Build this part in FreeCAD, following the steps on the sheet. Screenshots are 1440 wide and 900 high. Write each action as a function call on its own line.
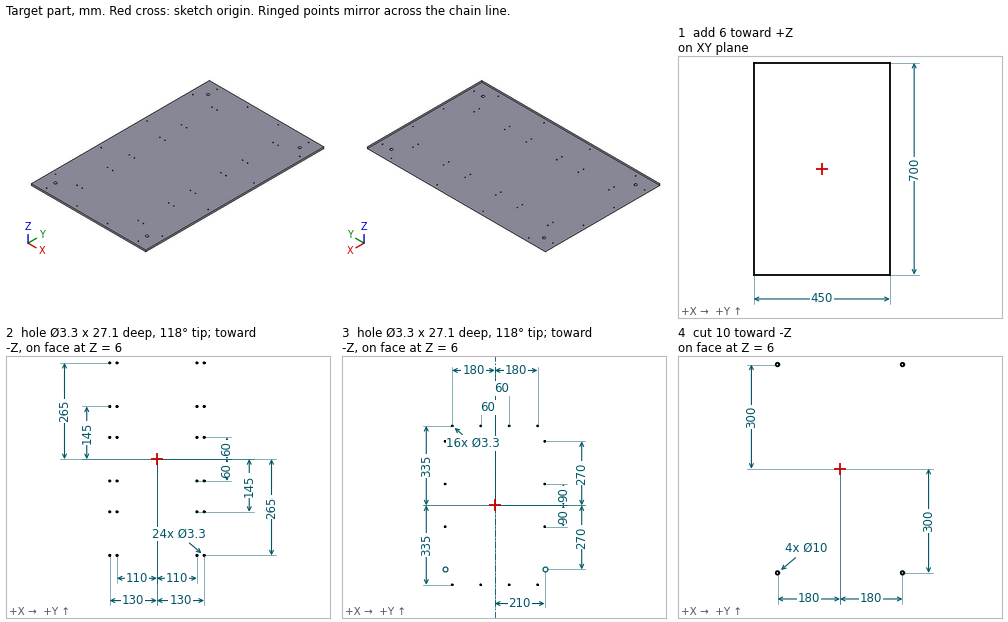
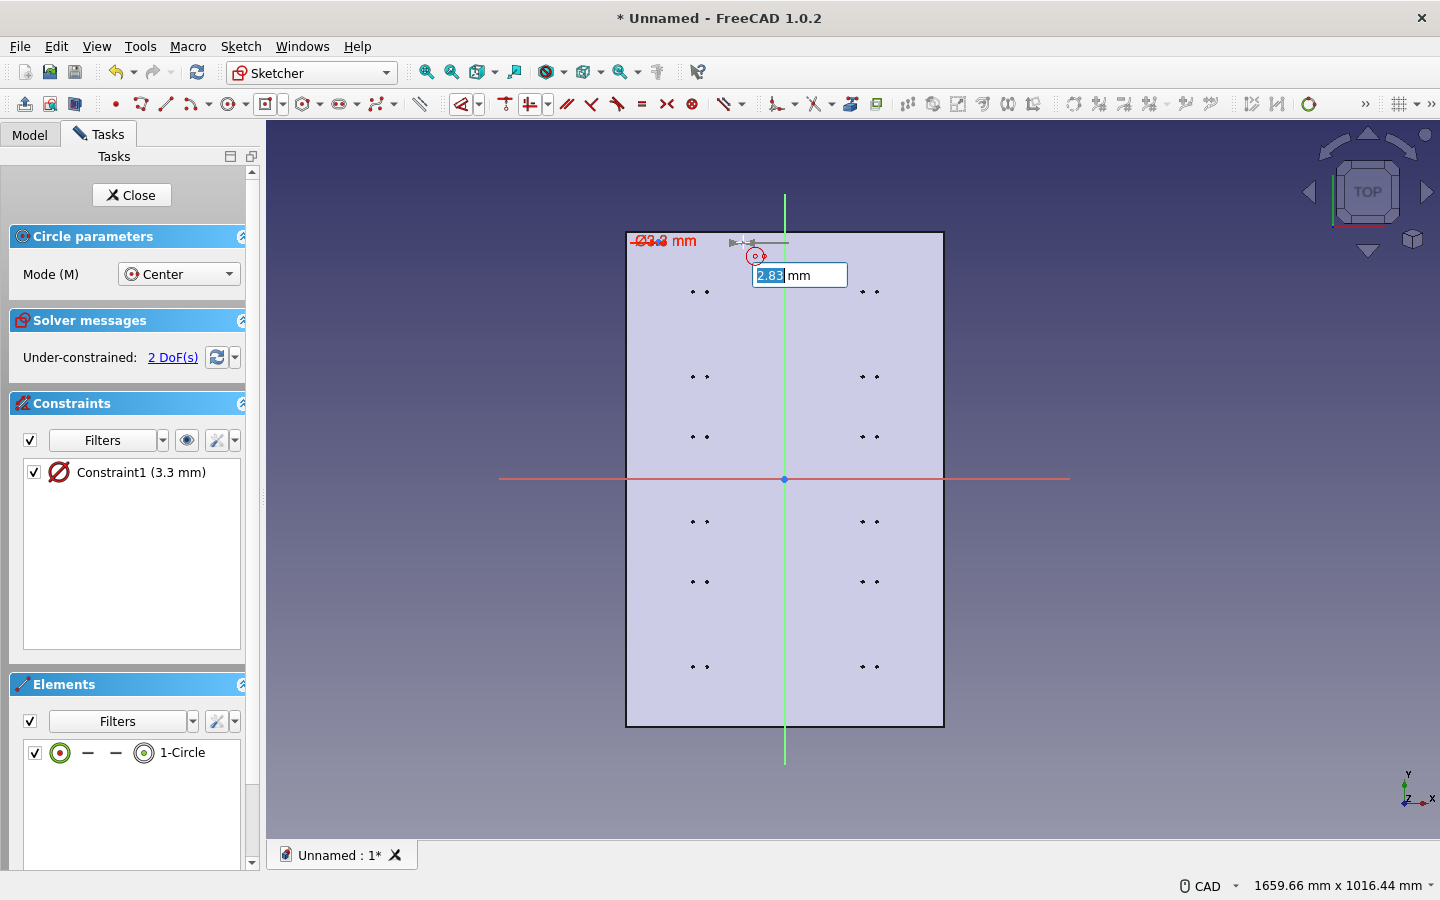
text(3.3)
key(Return)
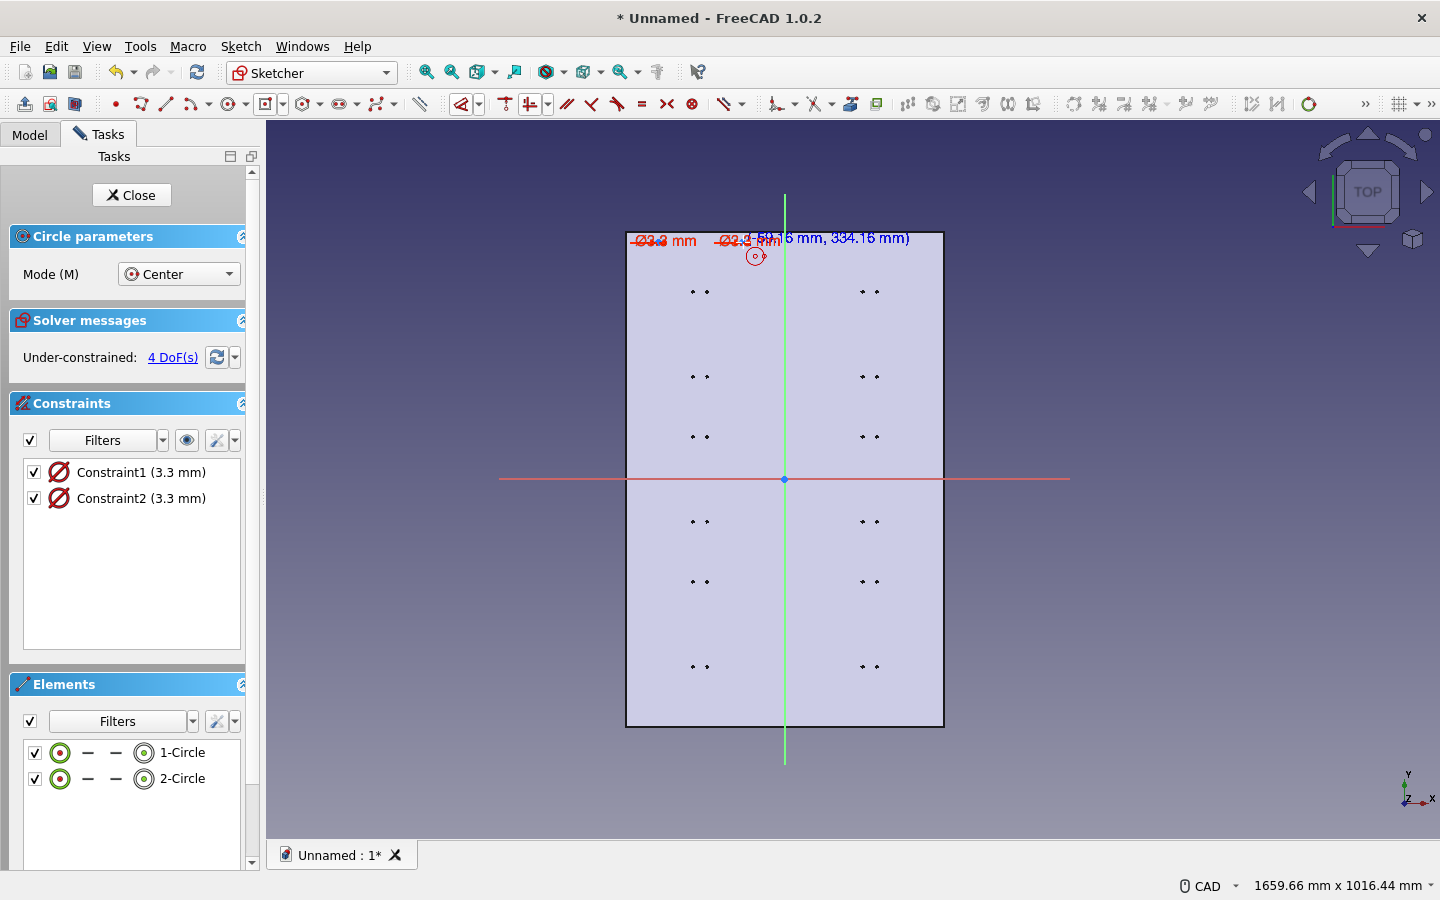
scroll(827, 242, up, 15)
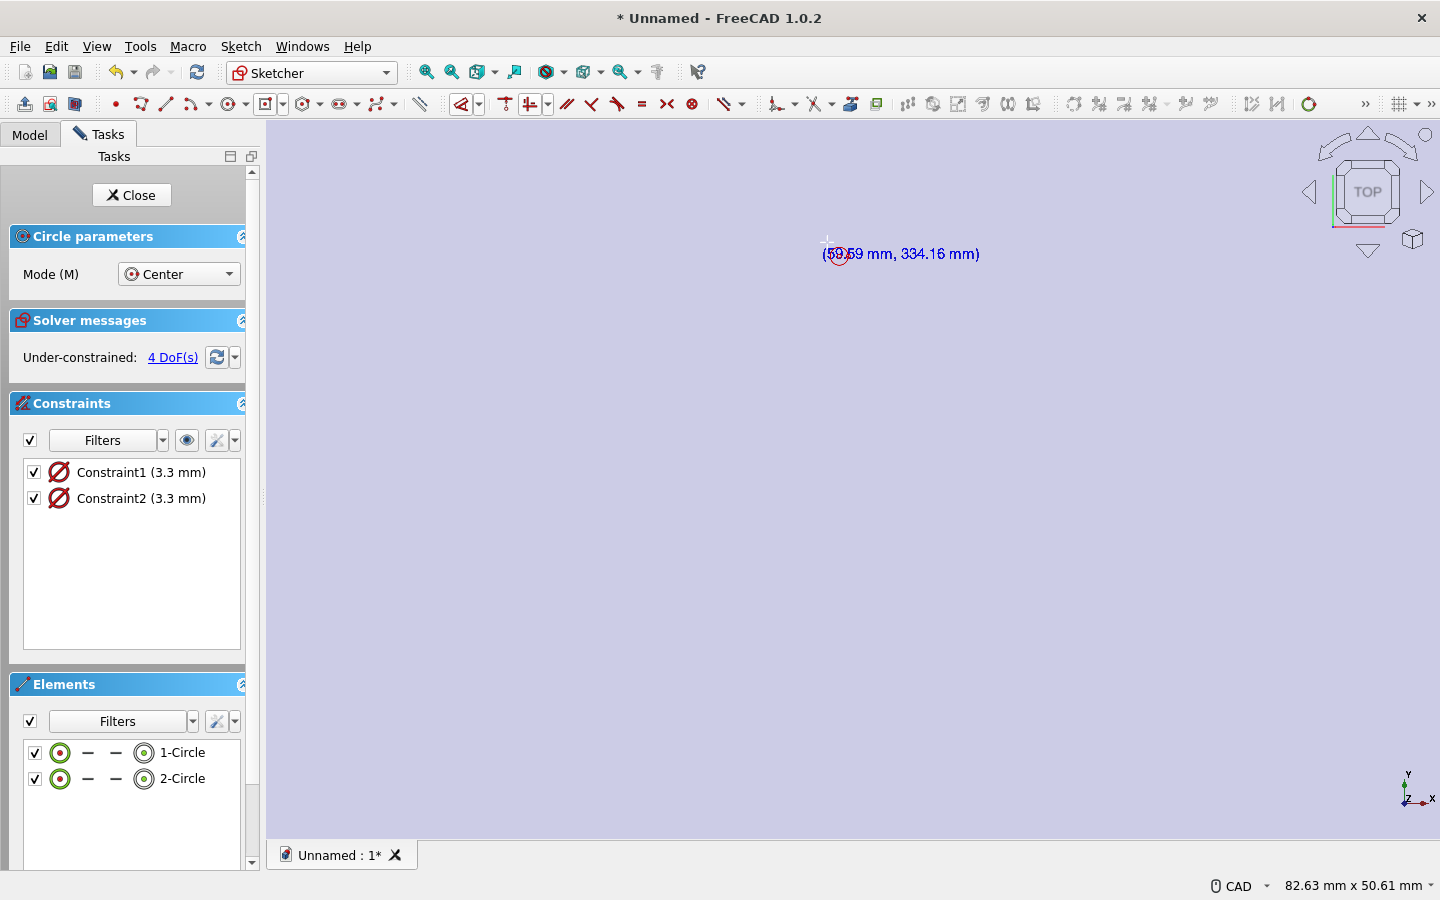
scroll(827, 242, down, 15)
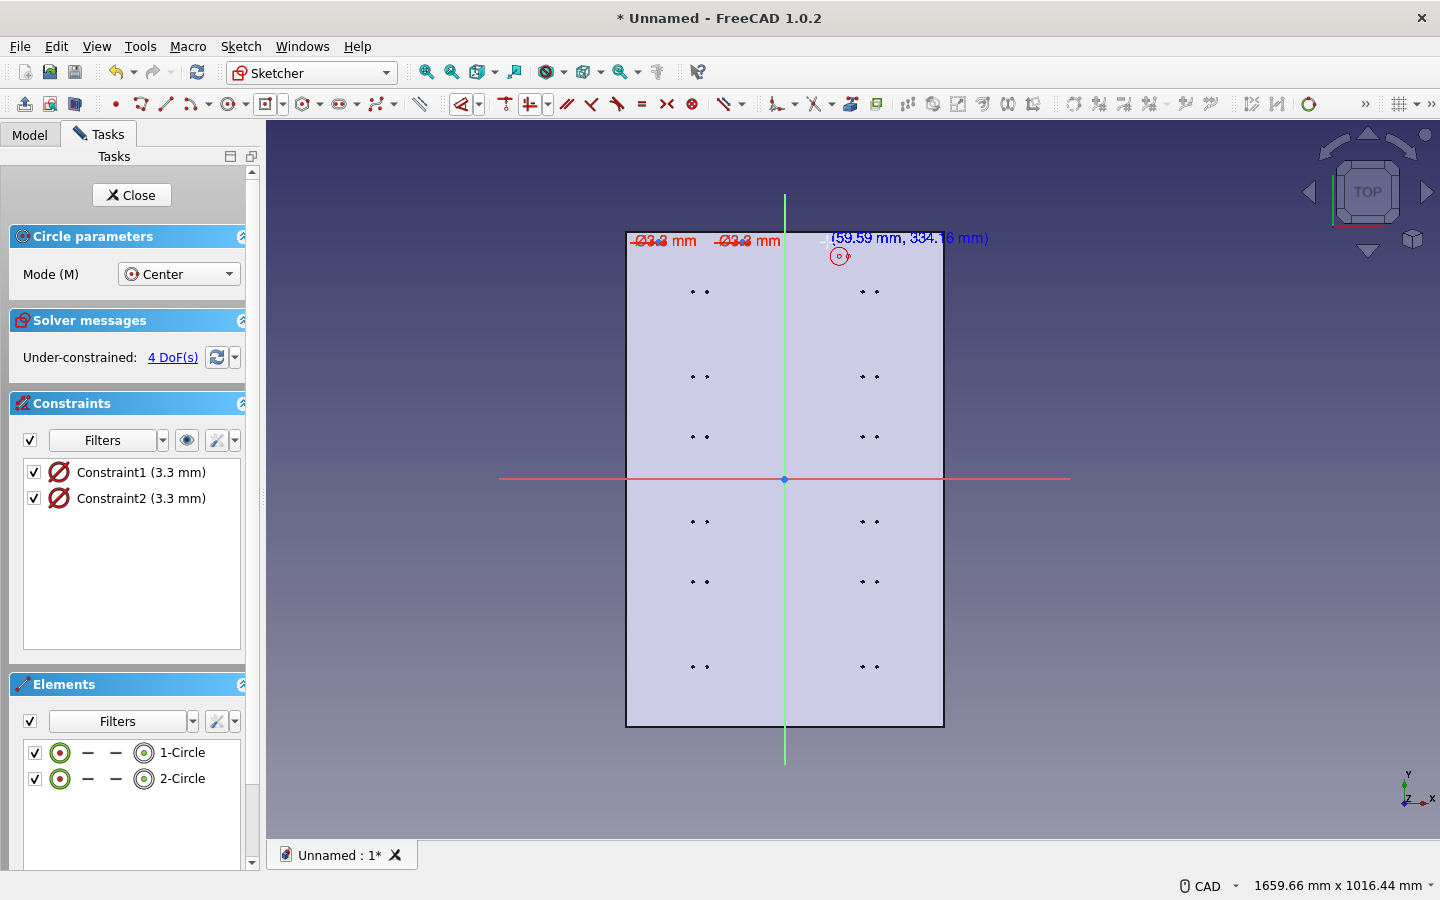
click(827, 242)
move(828, 242)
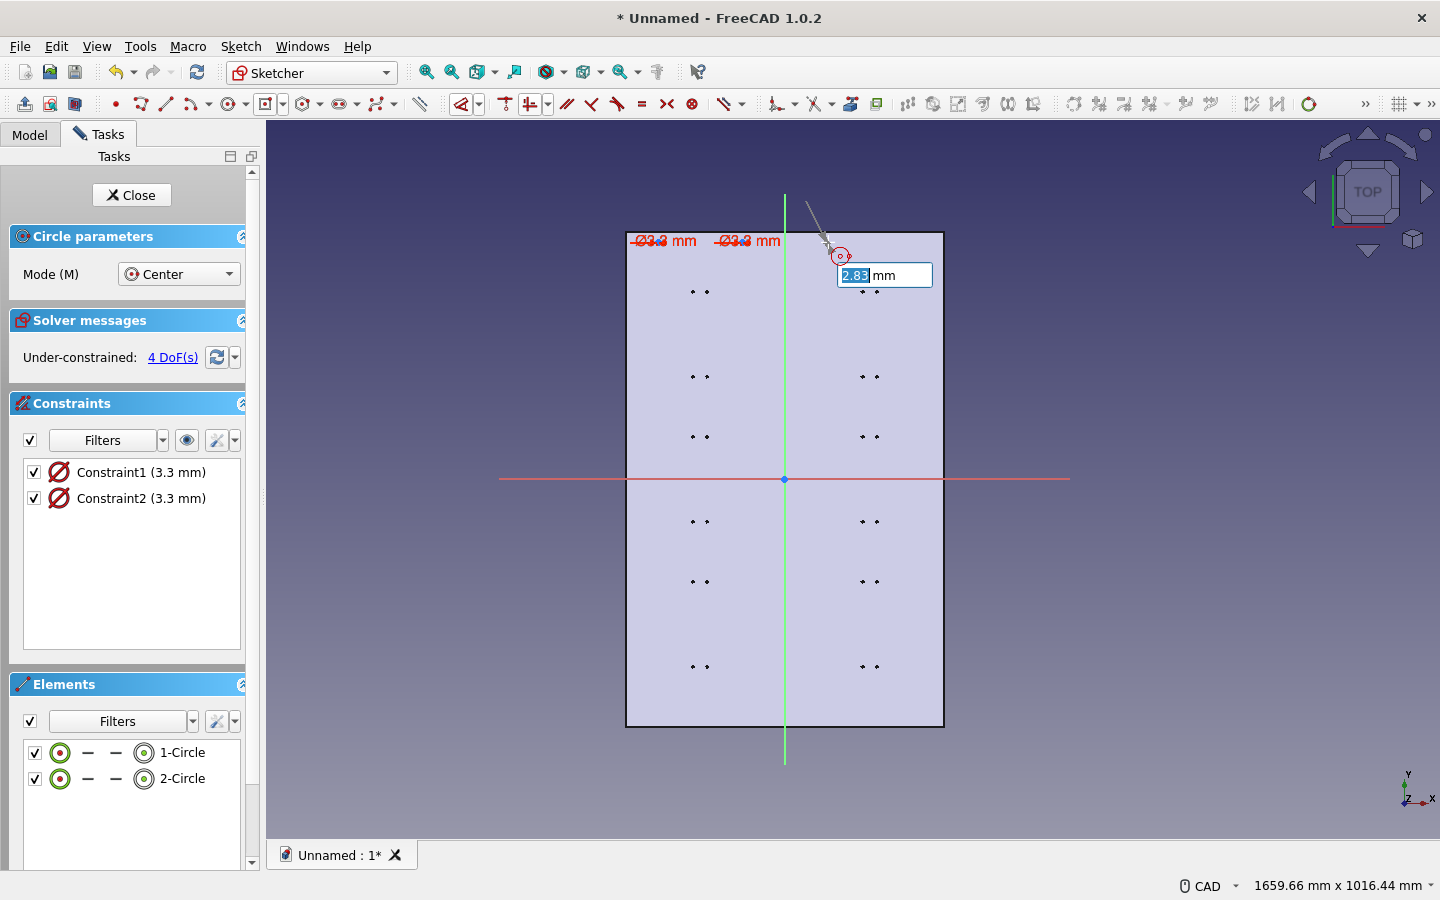
text(3.3)
key(Return)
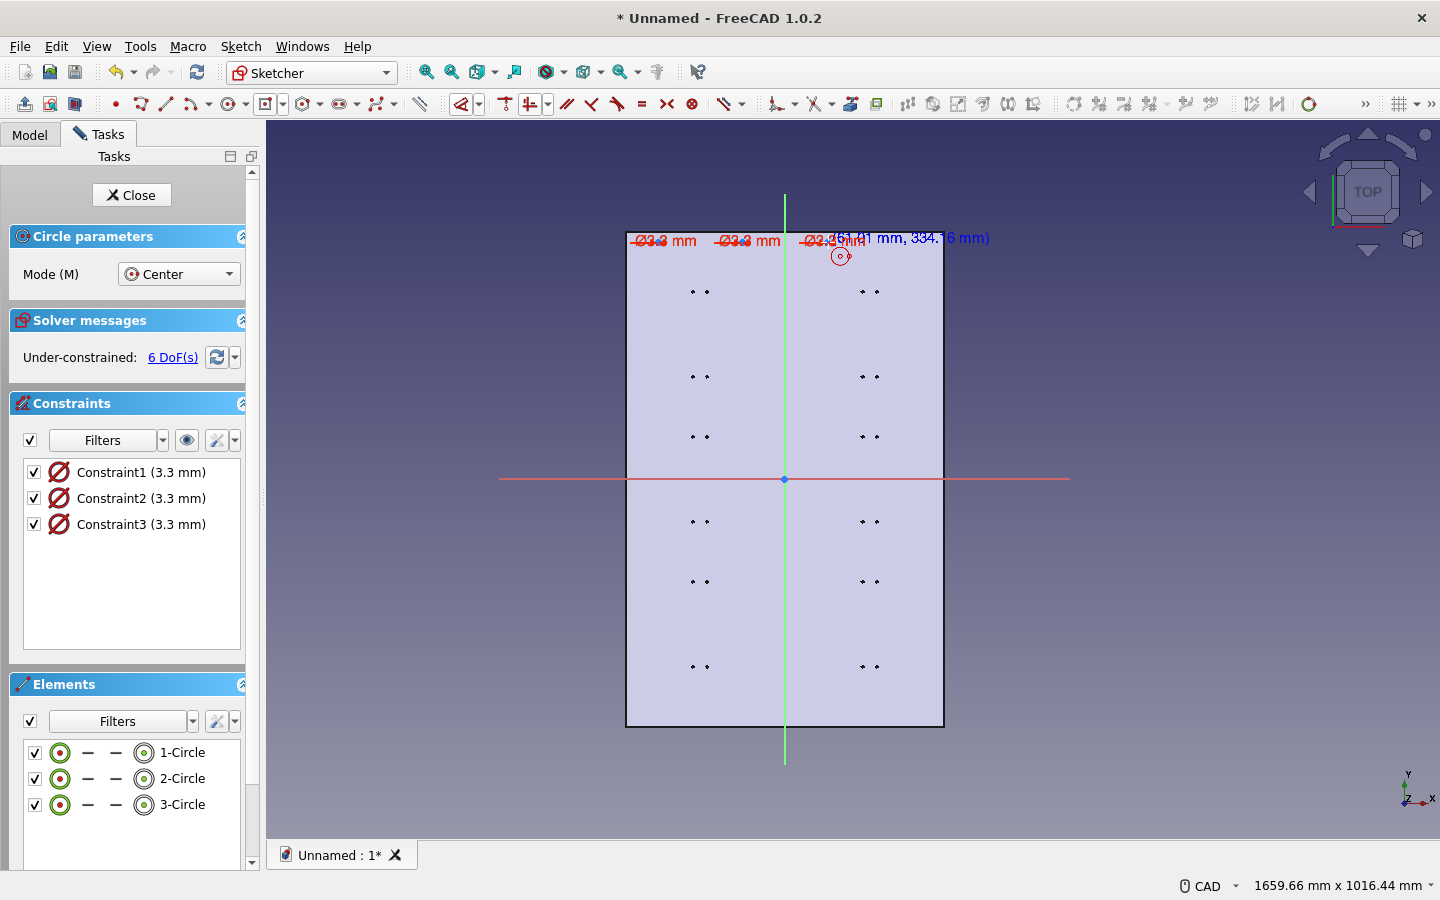
scroll(912, 242, up, 15)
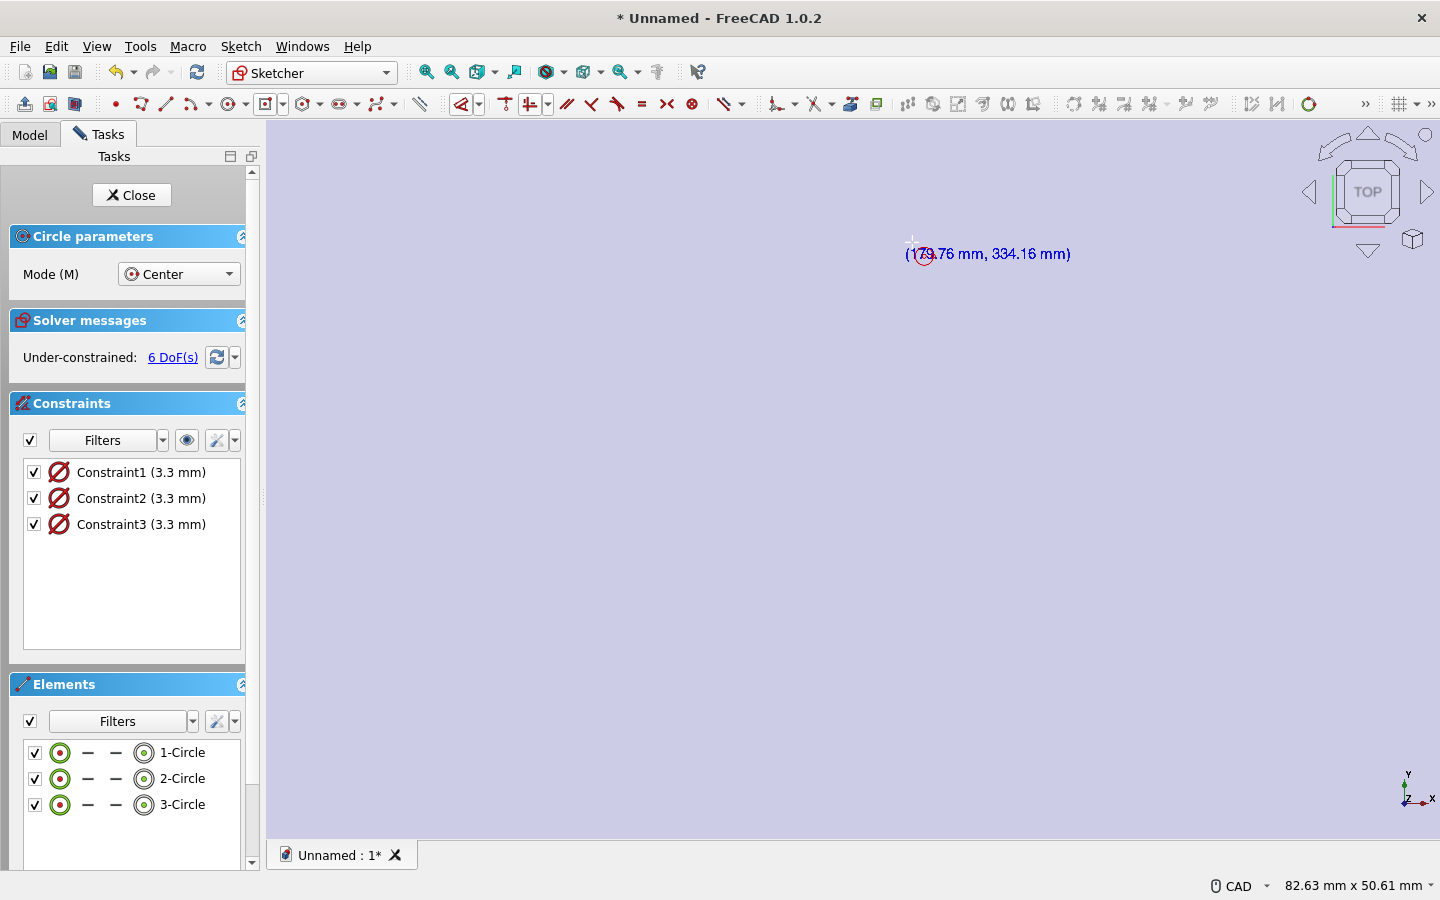
scroll(912, 242, down, 15)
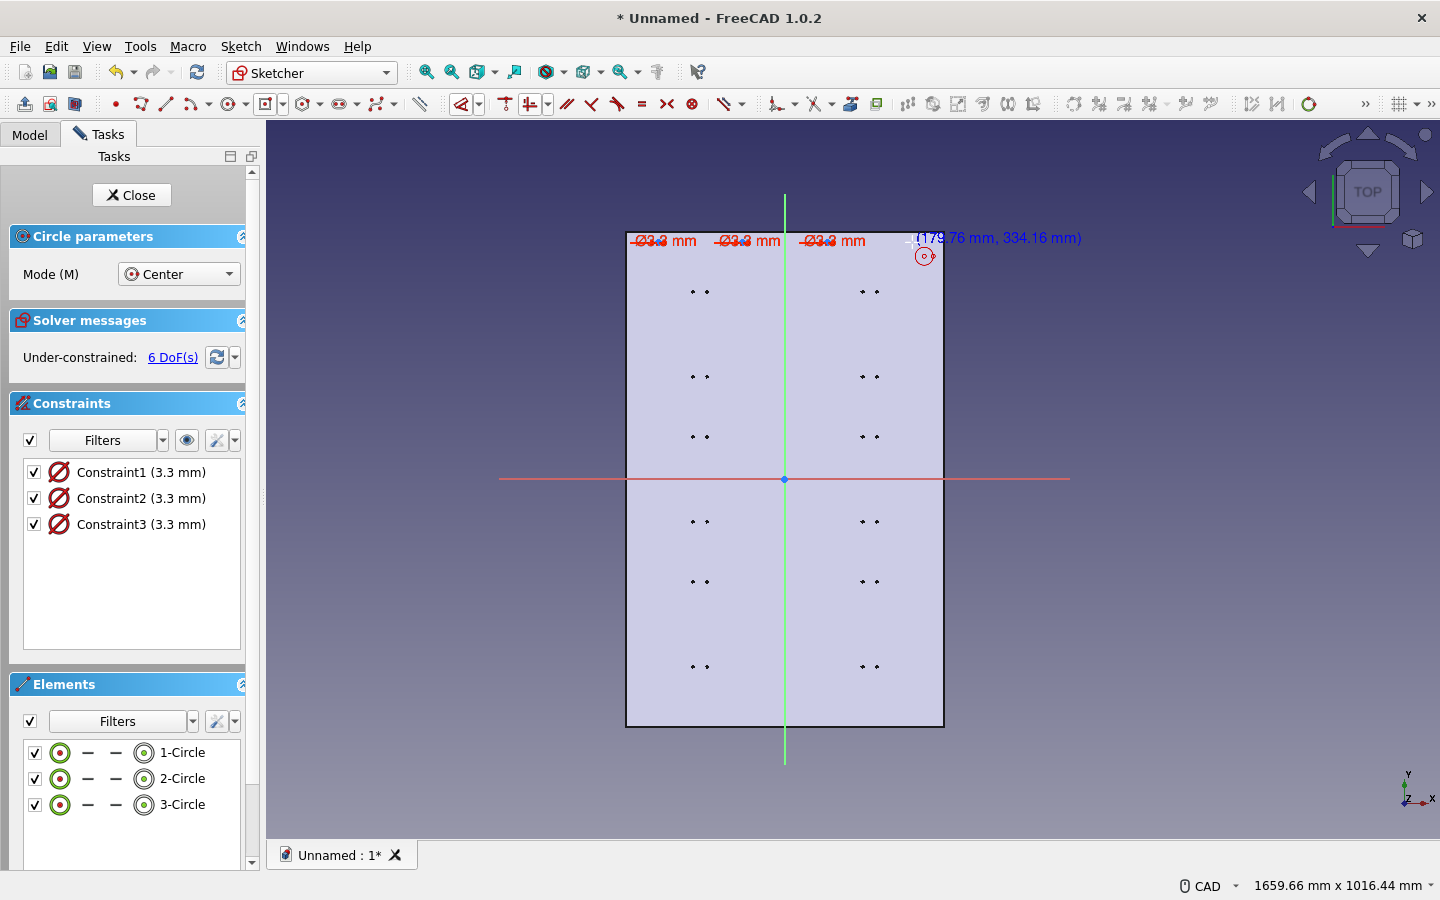
click(912, 242)
move(913, 242)